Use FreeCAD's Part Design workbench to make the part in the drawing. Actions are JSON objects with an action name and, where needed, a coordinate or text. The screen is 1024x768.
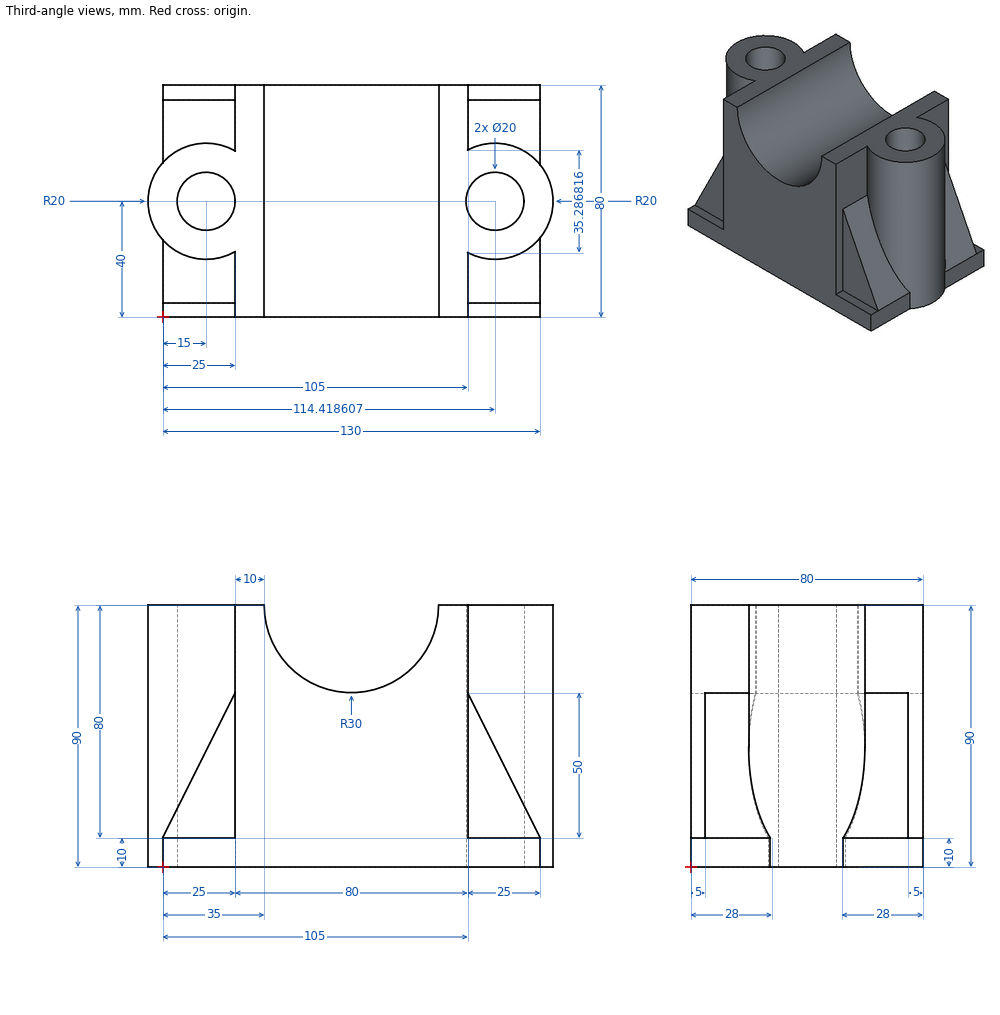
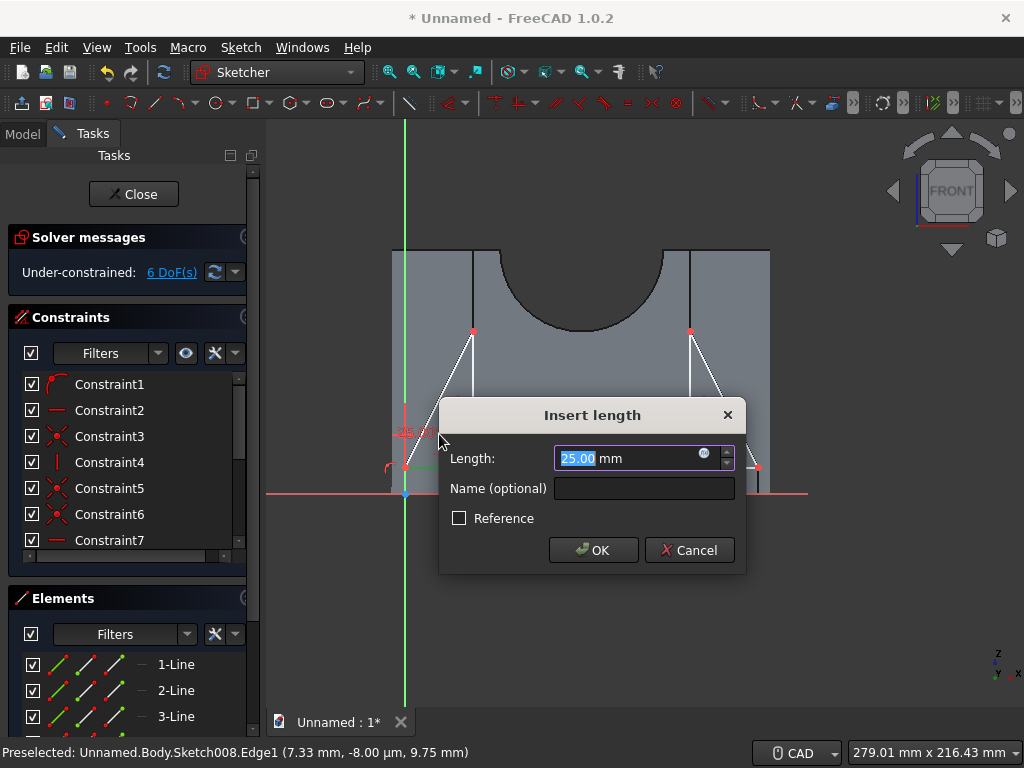
{"action": "type", "text": "25"}
{"action": "key", "text": "Return"}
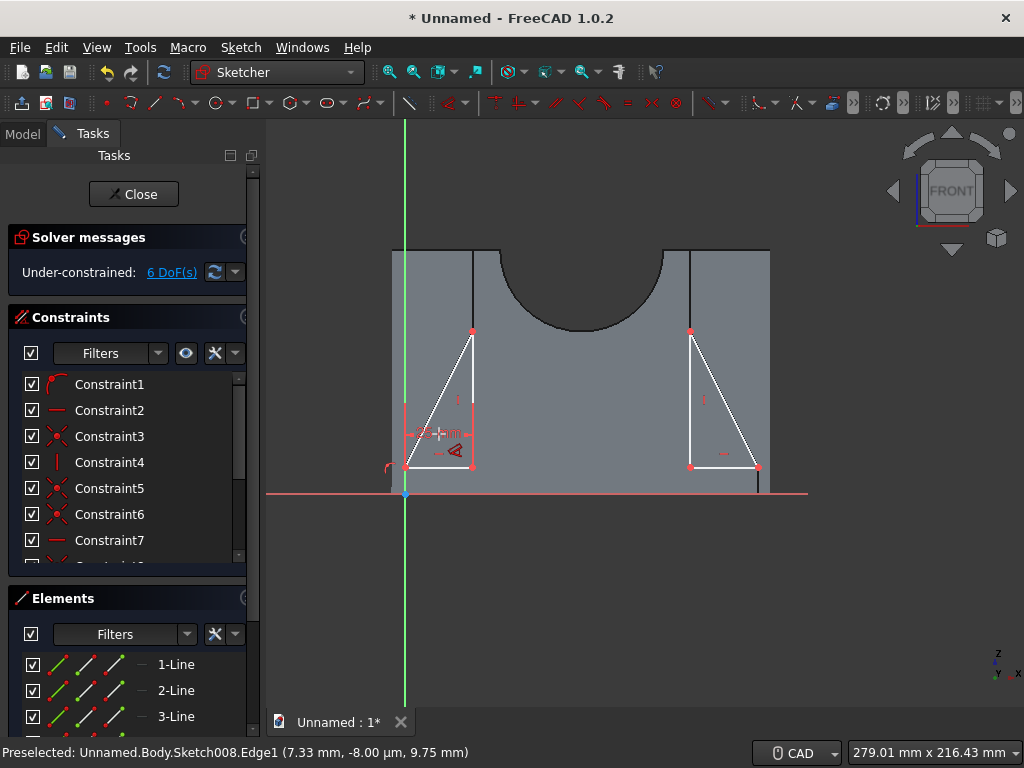
{"action": "left_click", "coordinate": [473, 427]}
{"action": "left_click", "coordinate": [439, 369]}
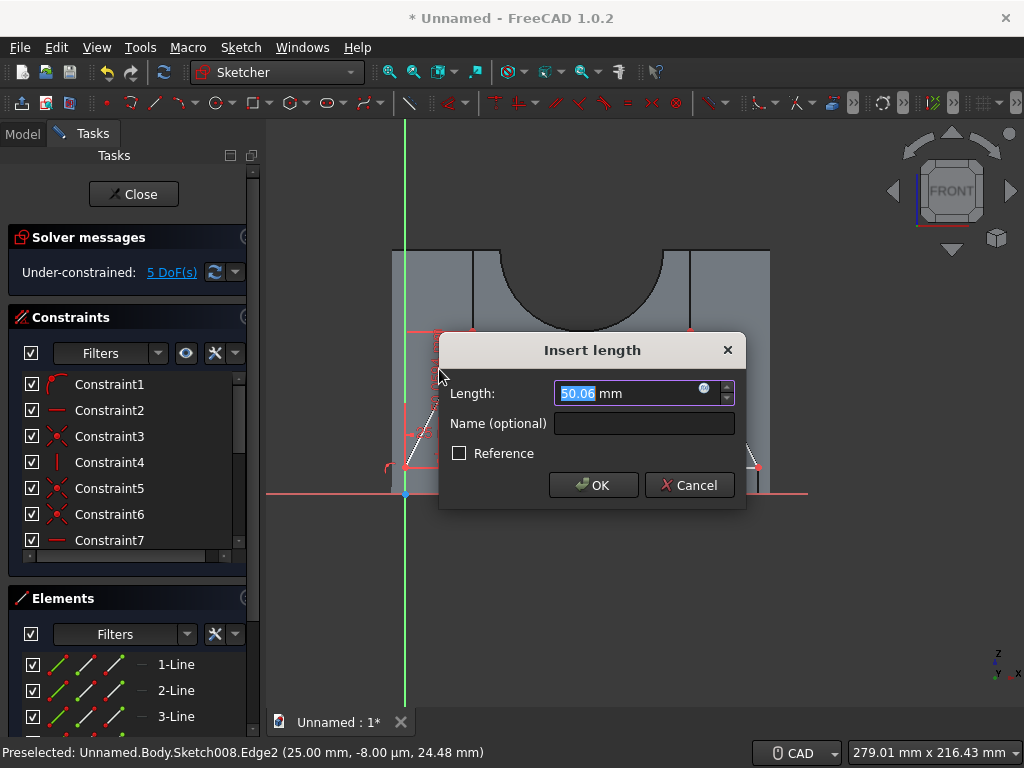
{"action": "type", "text": "50"}
{"action": "key", "text": "Return"}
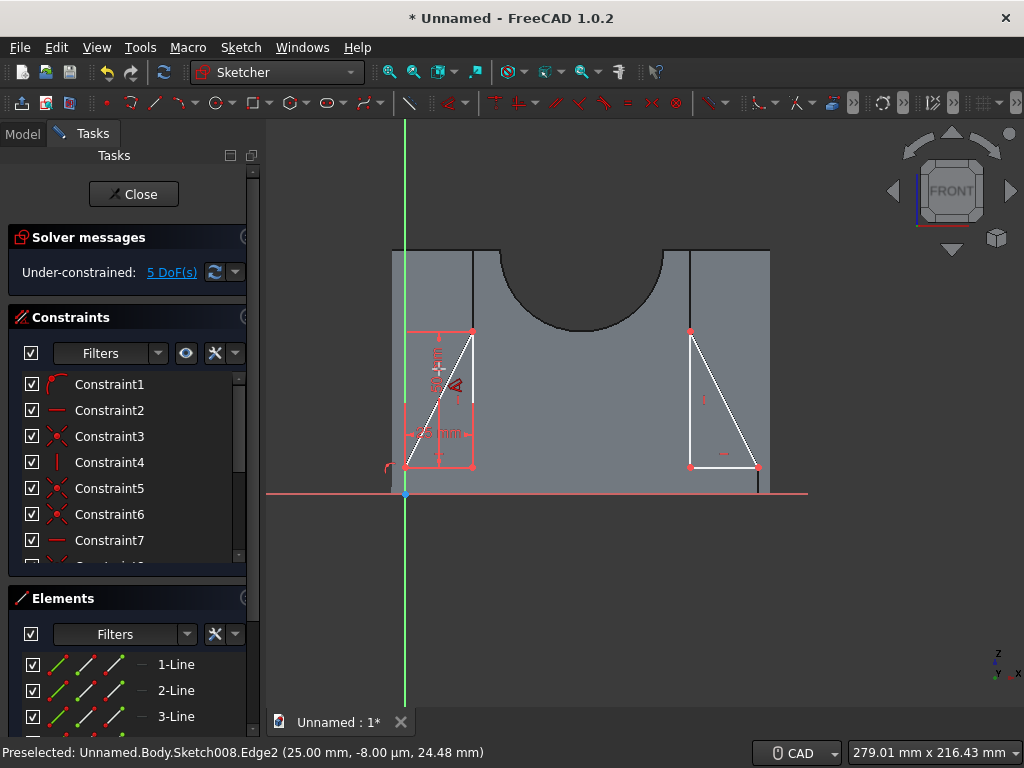
{"action": "left_click", "coordinate": [710, 468]}
{"action": "left_click", "coordinate": [724, 434]}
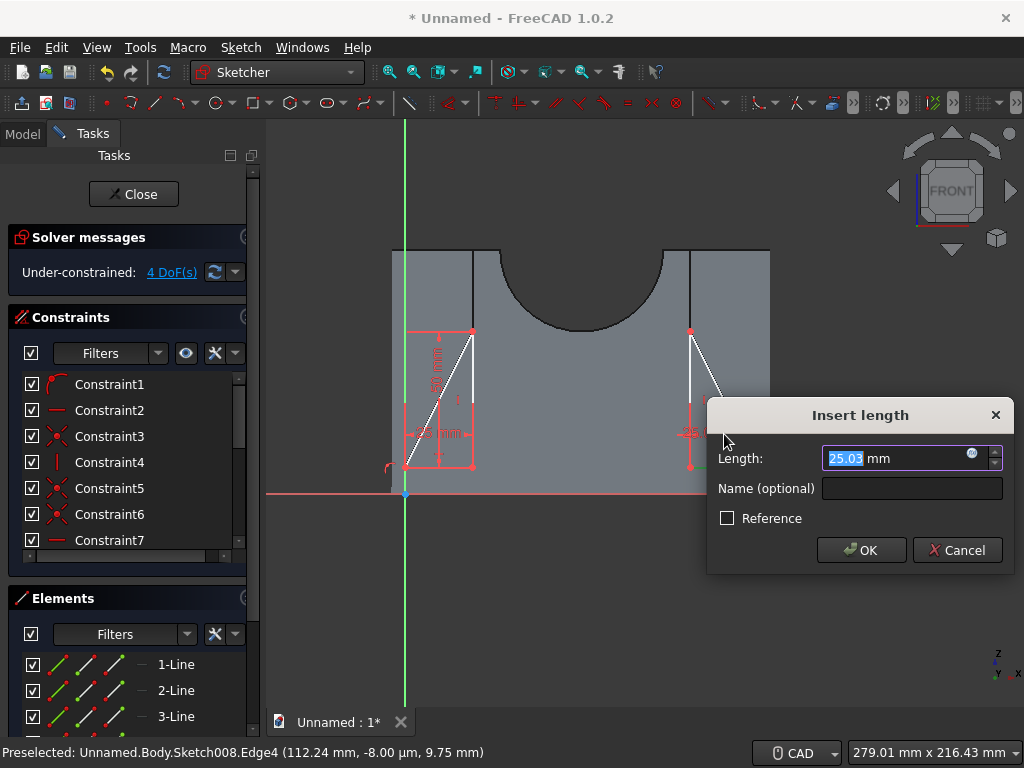
{"action": "type", "text": "25"}
{"action": "key", "text": "Return"}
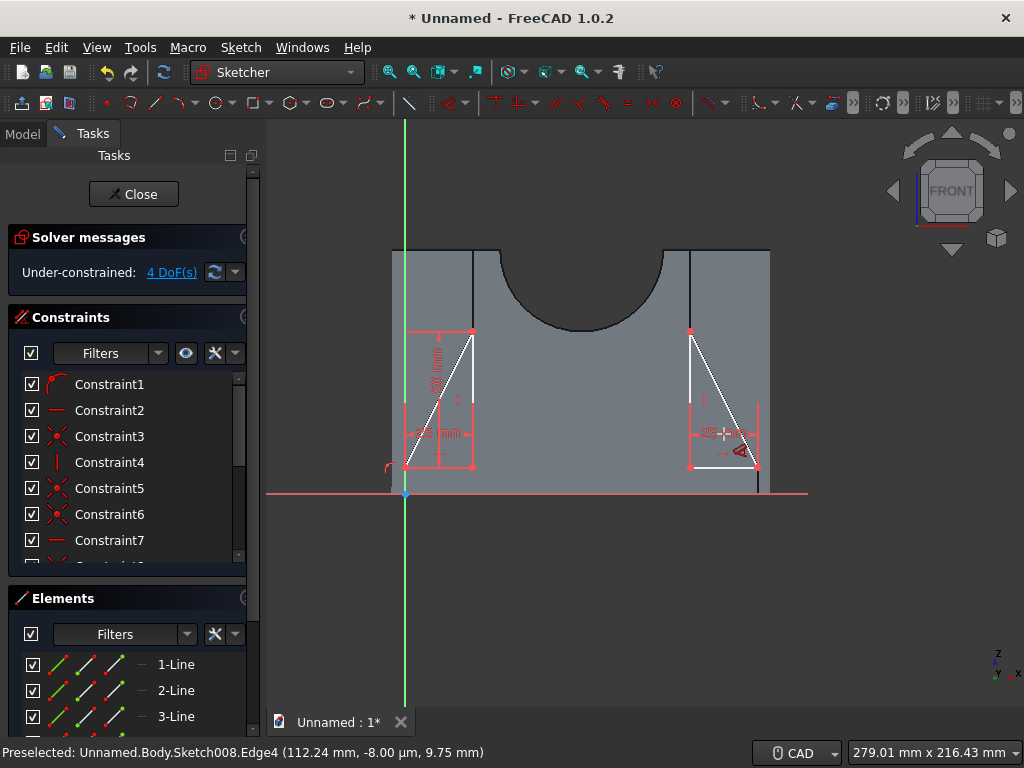
{"action": "left_click", "coordinate": [690, 373]}
{"action": "left_click", "coordinate": [724, 369]}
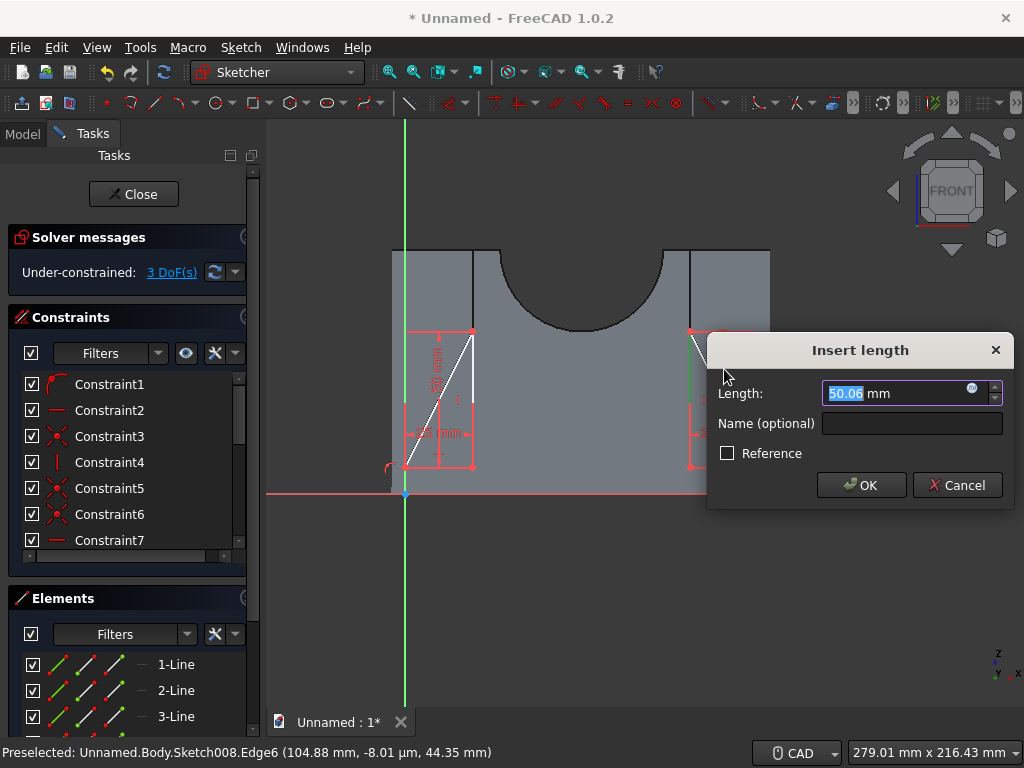
{"action": "type", "text": "50"}
{"action": "key", "text": "Return"}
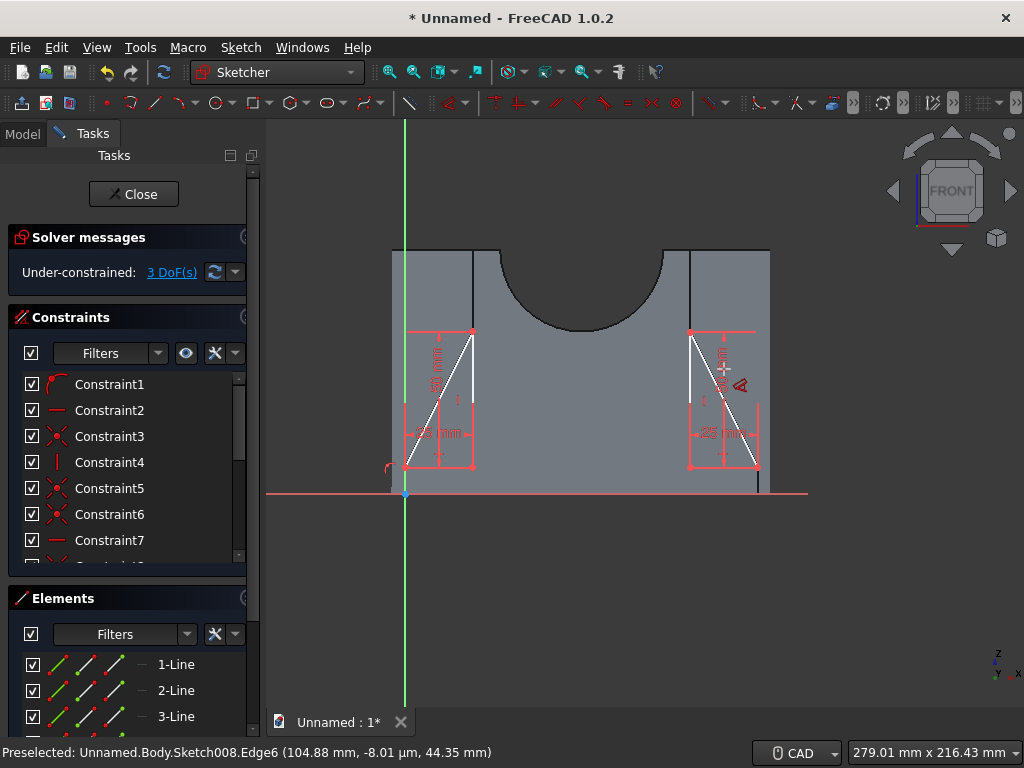
{"action": "scroll", "coordinate": [405, 468], "scroll_direction": "up", "scroll_amount": 2}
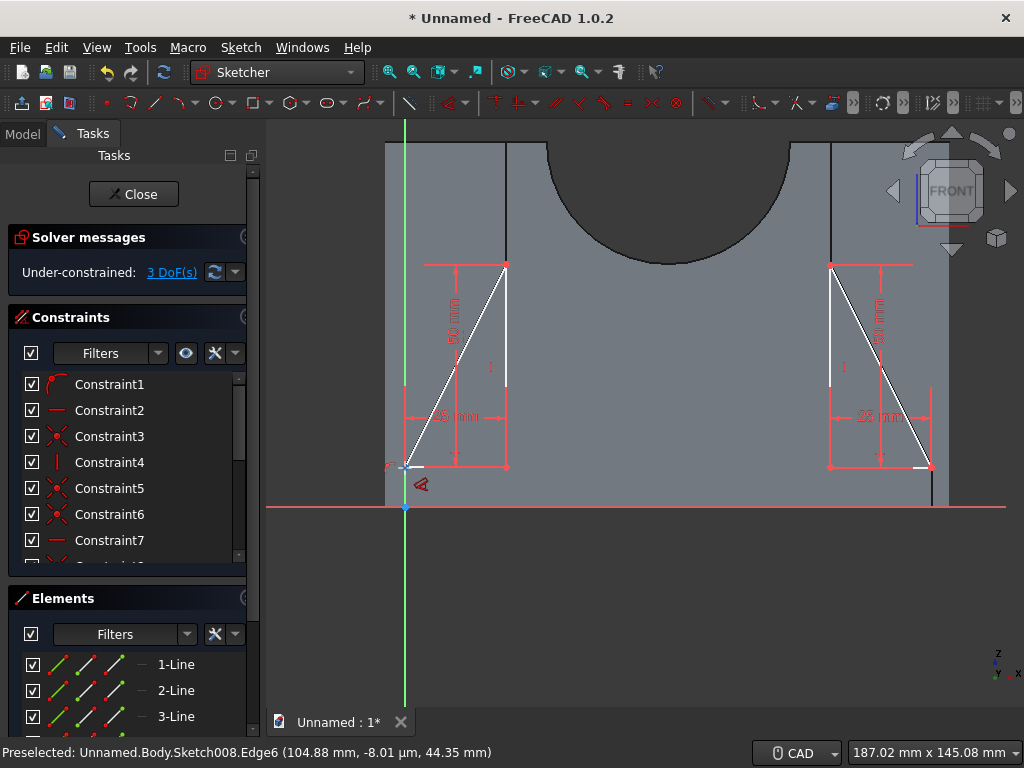
{"action": "left_click", "coordinate": [405, 467]}
{"action": "left_click", "coordinate": [371, 487]}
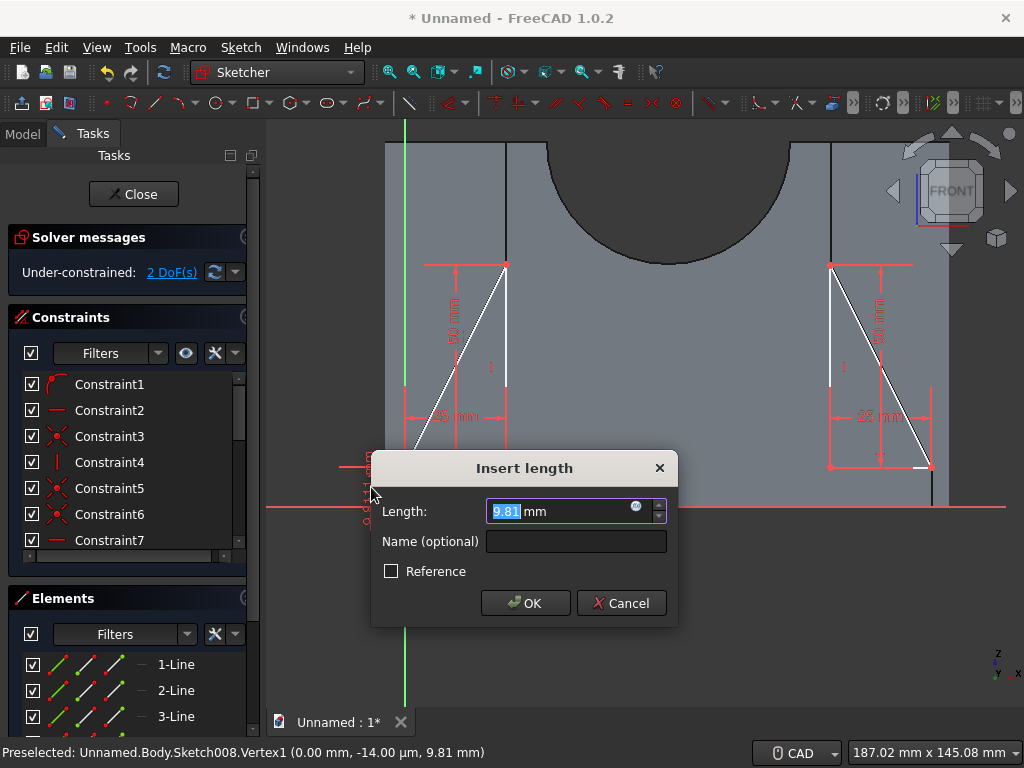
{"action": "type", "text": "10"}
{"action": "key", "text": "Return"}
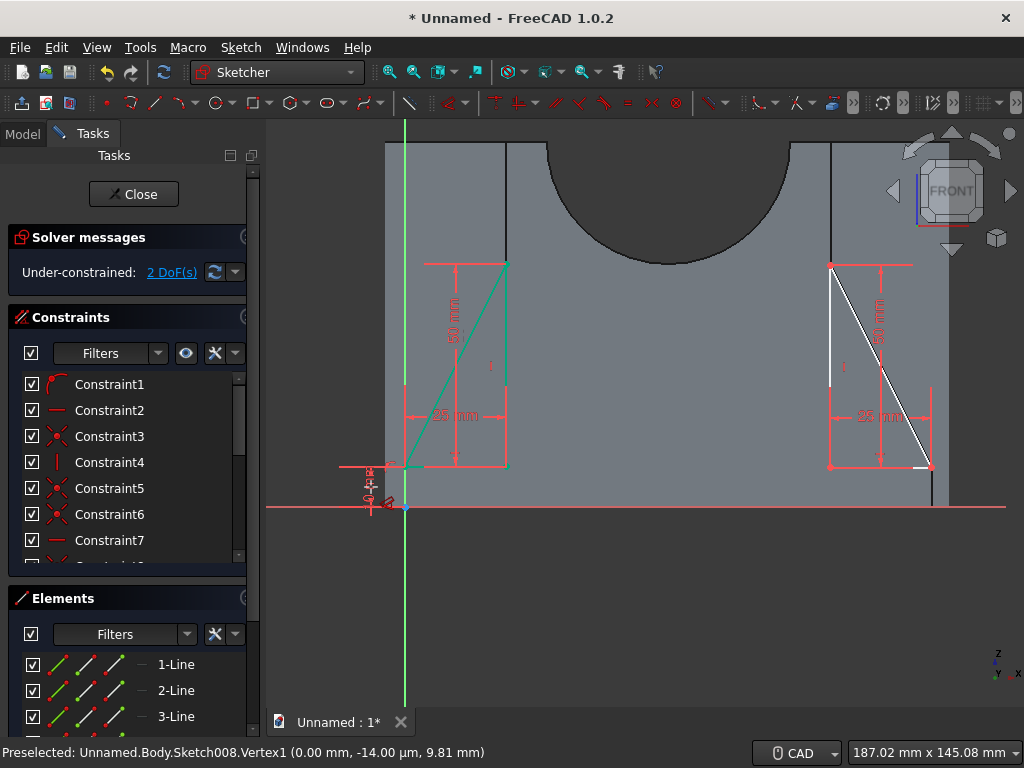
{"action": "left_click", "coordinate": [830, 468]}
{"action": "left_click", "coordinate": [299, 487]}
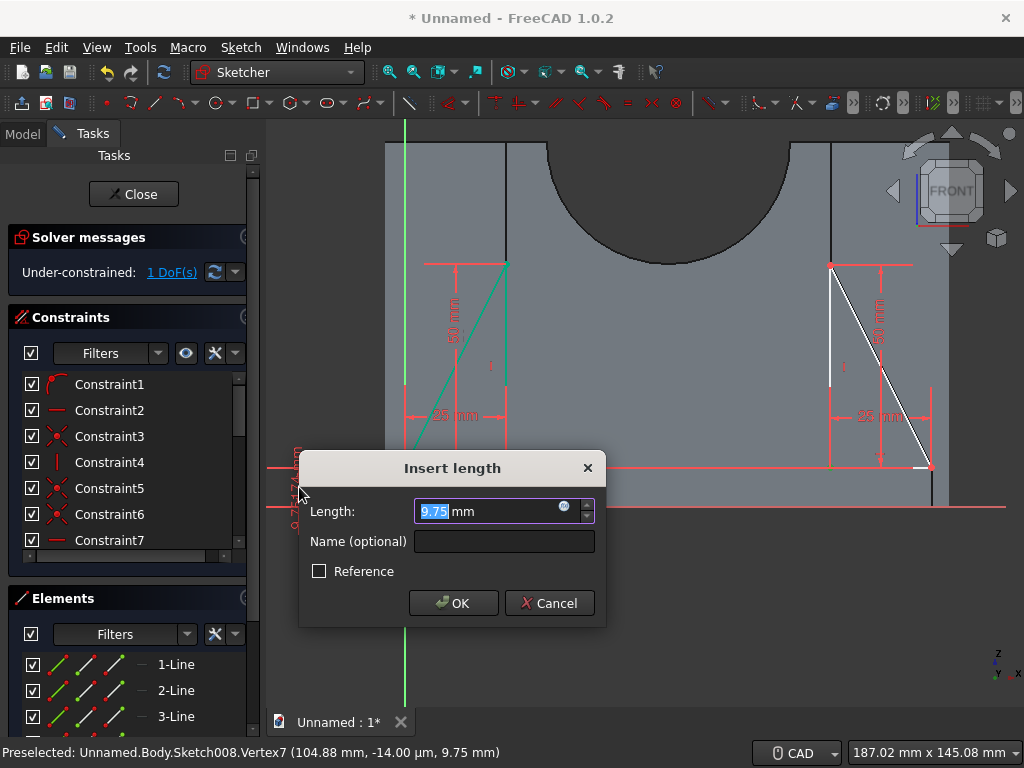
{"action": "type", "text": "10"}
{"action": "key", "text": "Return"}